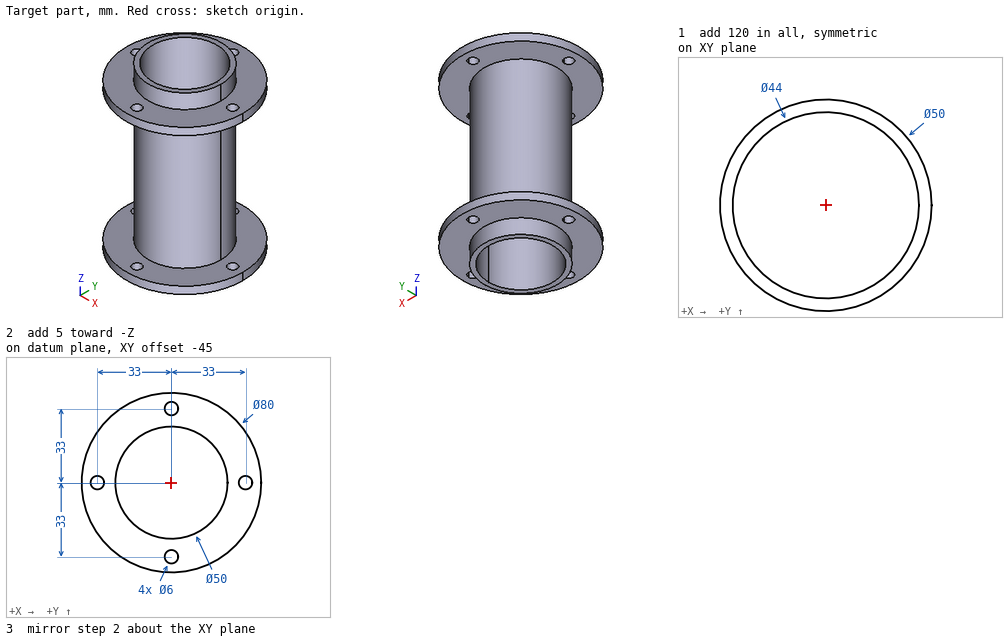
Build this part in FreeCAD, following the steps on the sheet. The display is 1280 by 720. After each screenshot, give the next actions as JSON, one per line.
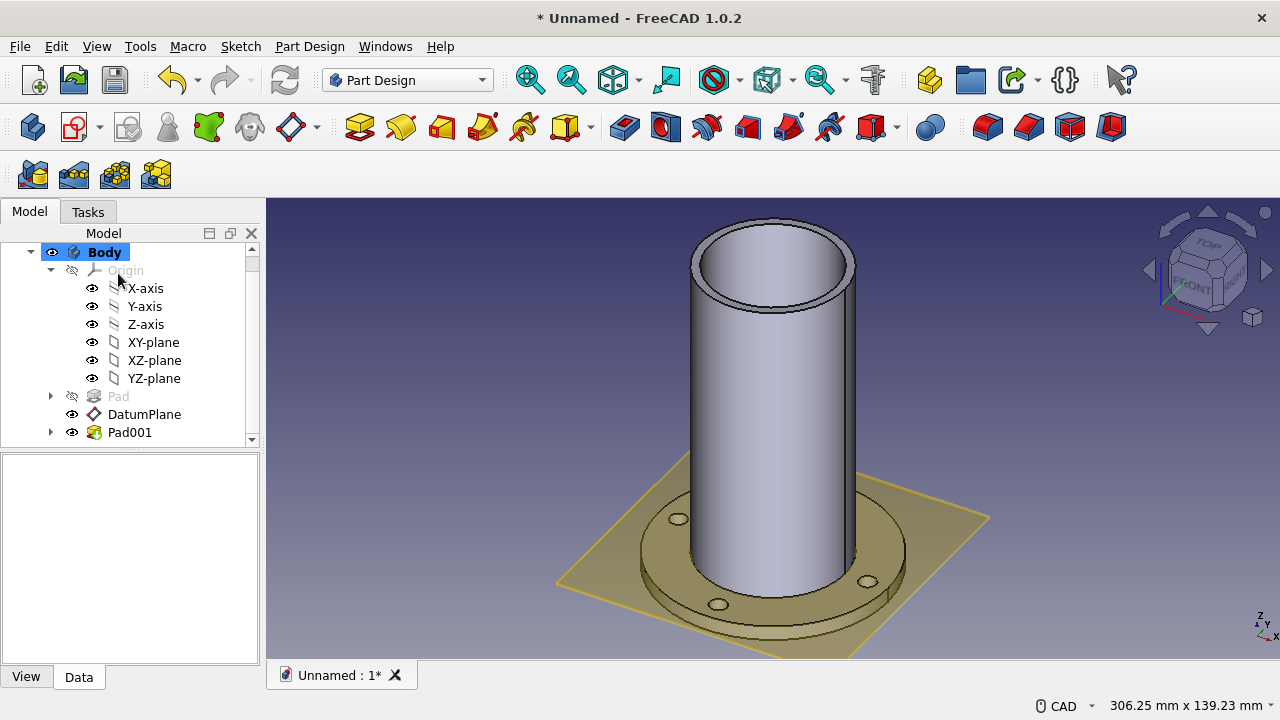
{"action": "left_click", "coordinate": [117, 414]}
{"action": "key", "text": "space"}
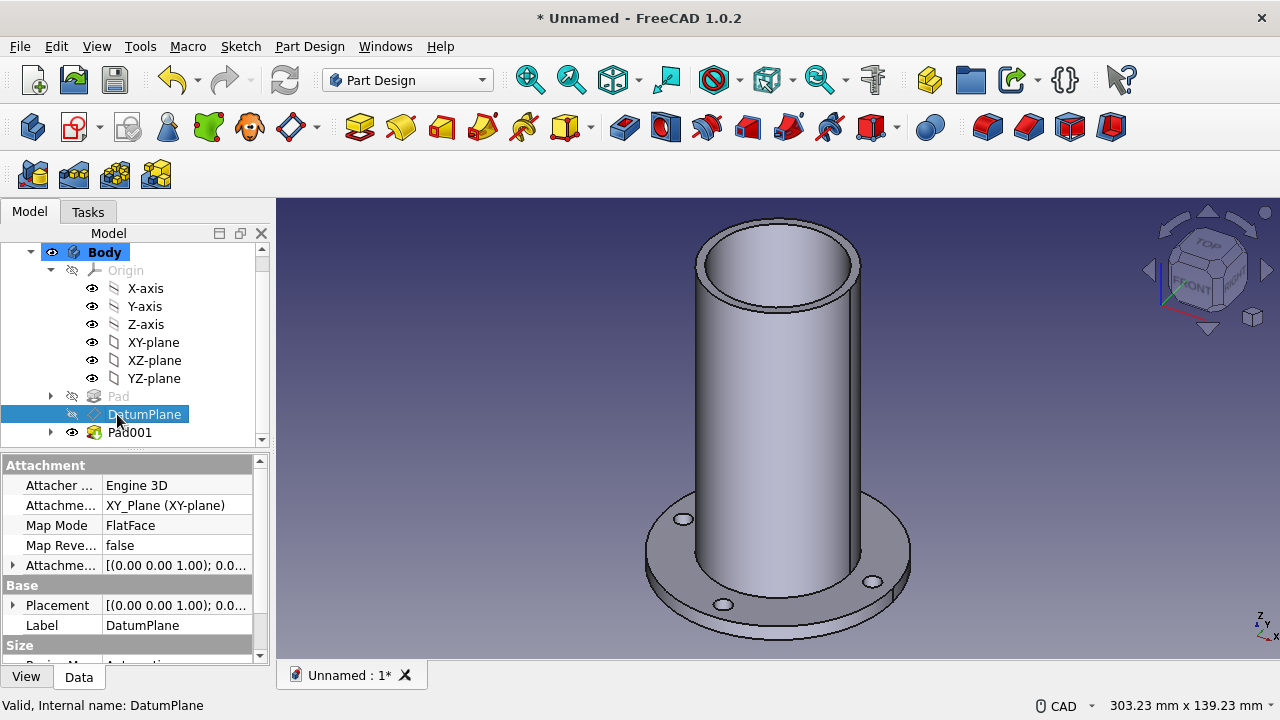
{"action": "left_click", "coordinate": [531, 80]}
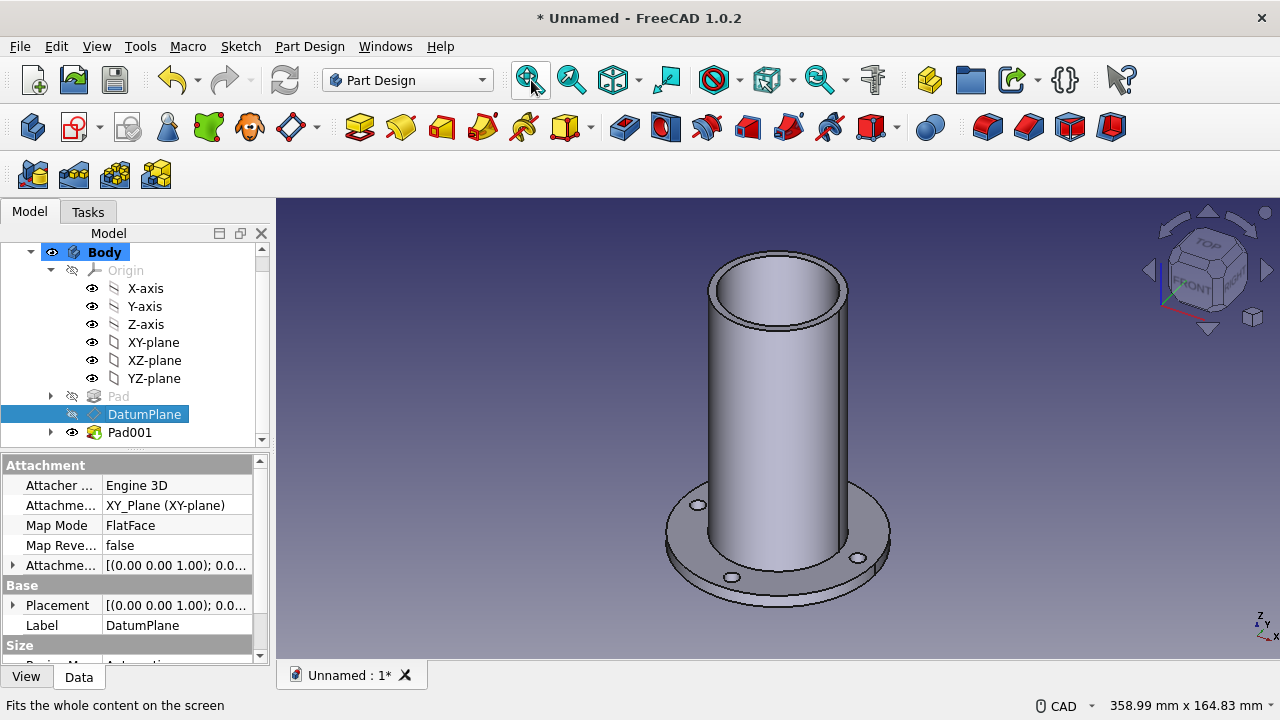
{"action": "left_click", "coordinate": [117, 432]}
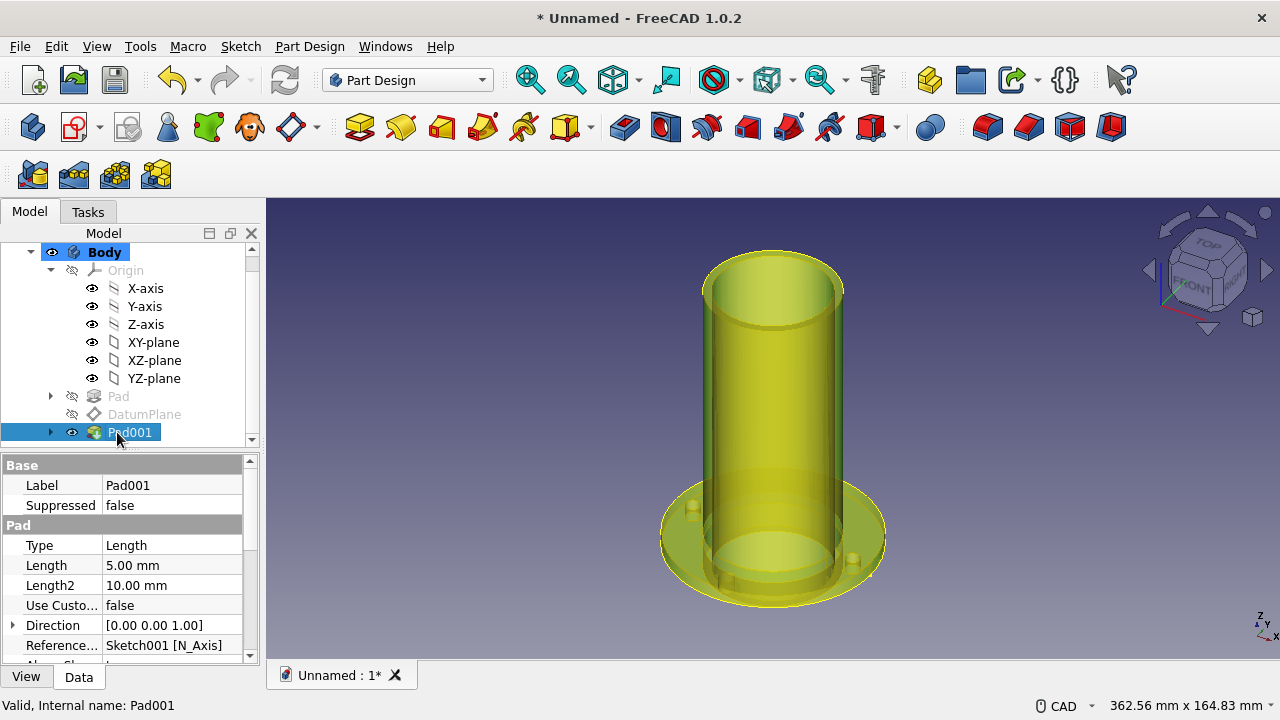
{"action": "left_click", "coordinate": [33, 174]}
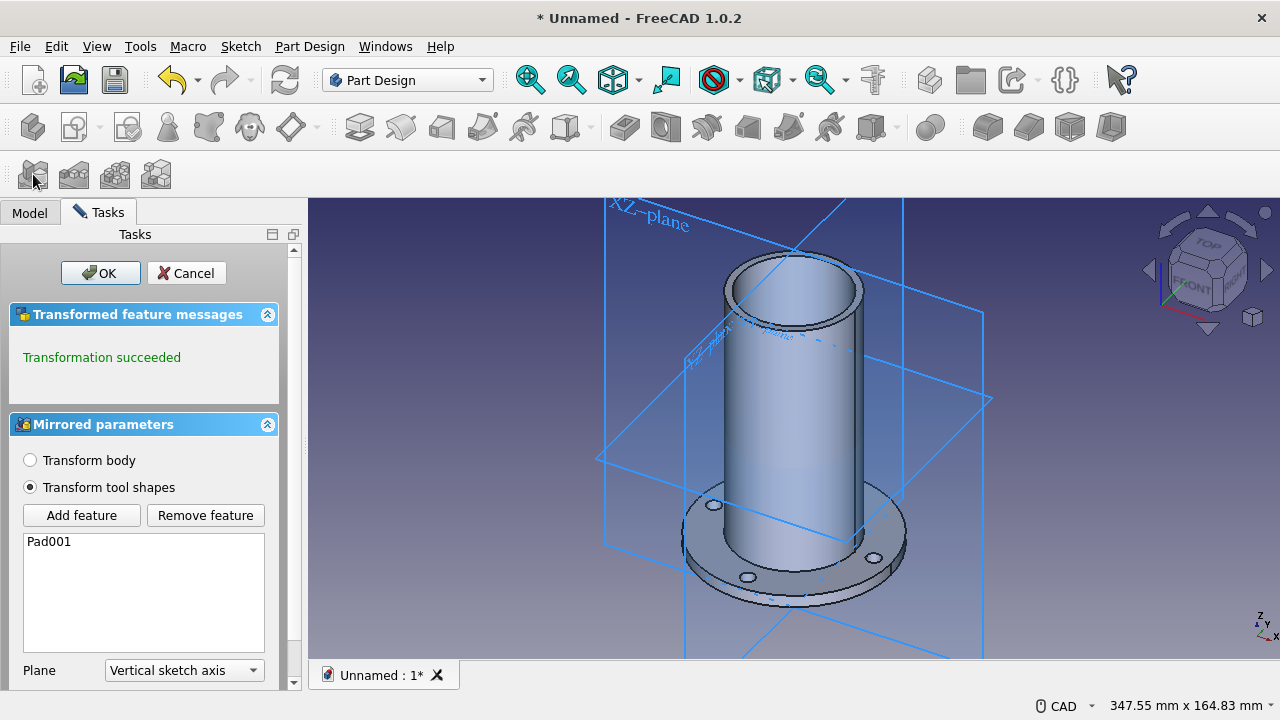
{"action": "left_click", "coordinate": [185, 670]}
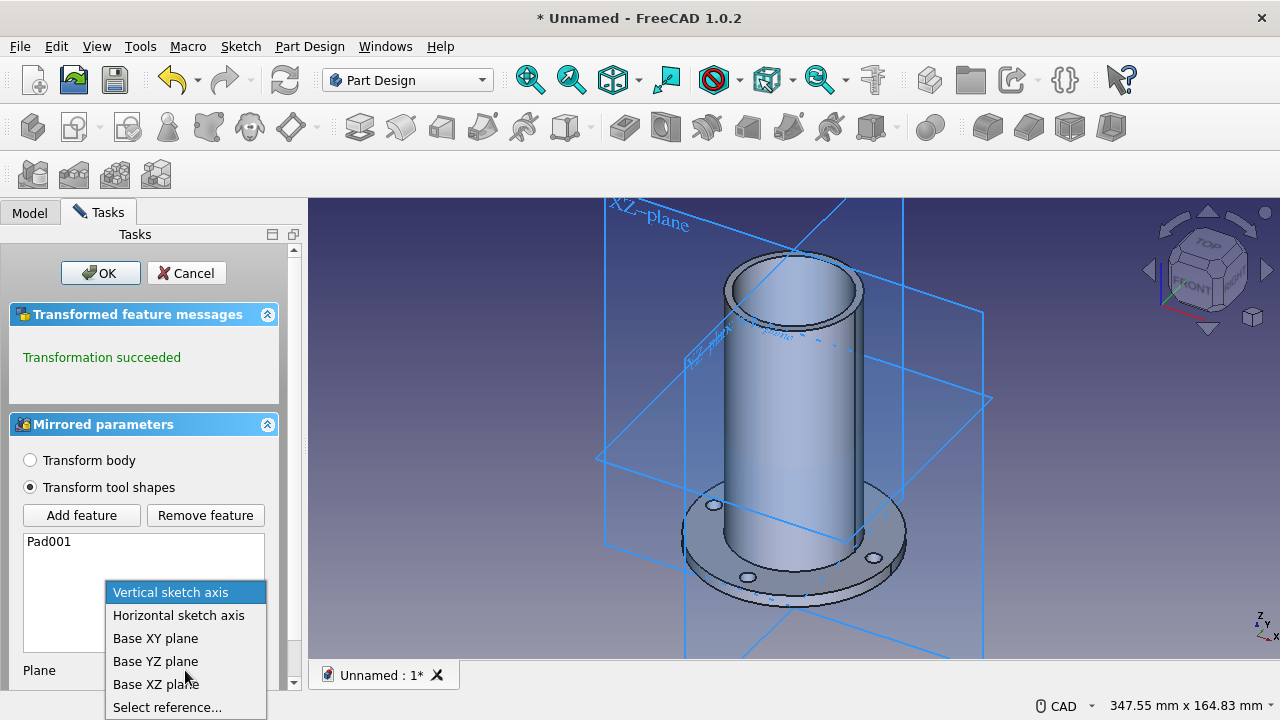
{"action": "left_click", "coordinate": [184, 638]}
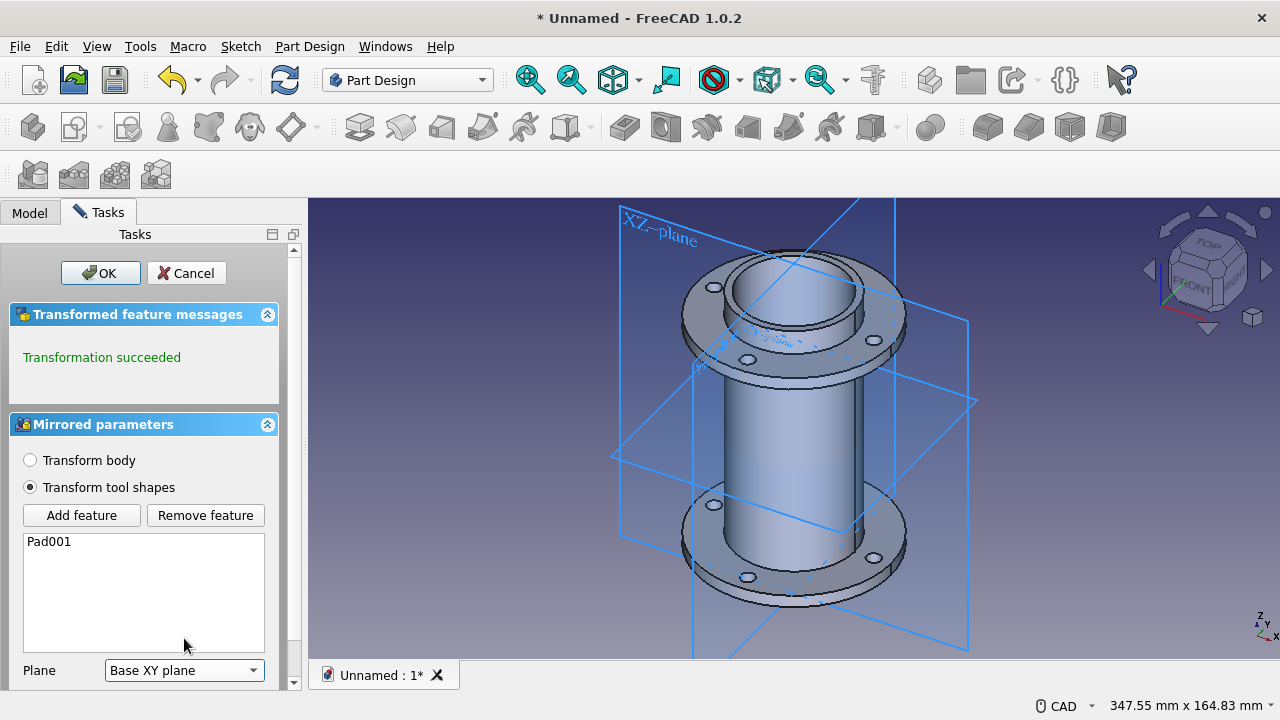
{"action": "left_click", "coordinate": [101, 273]}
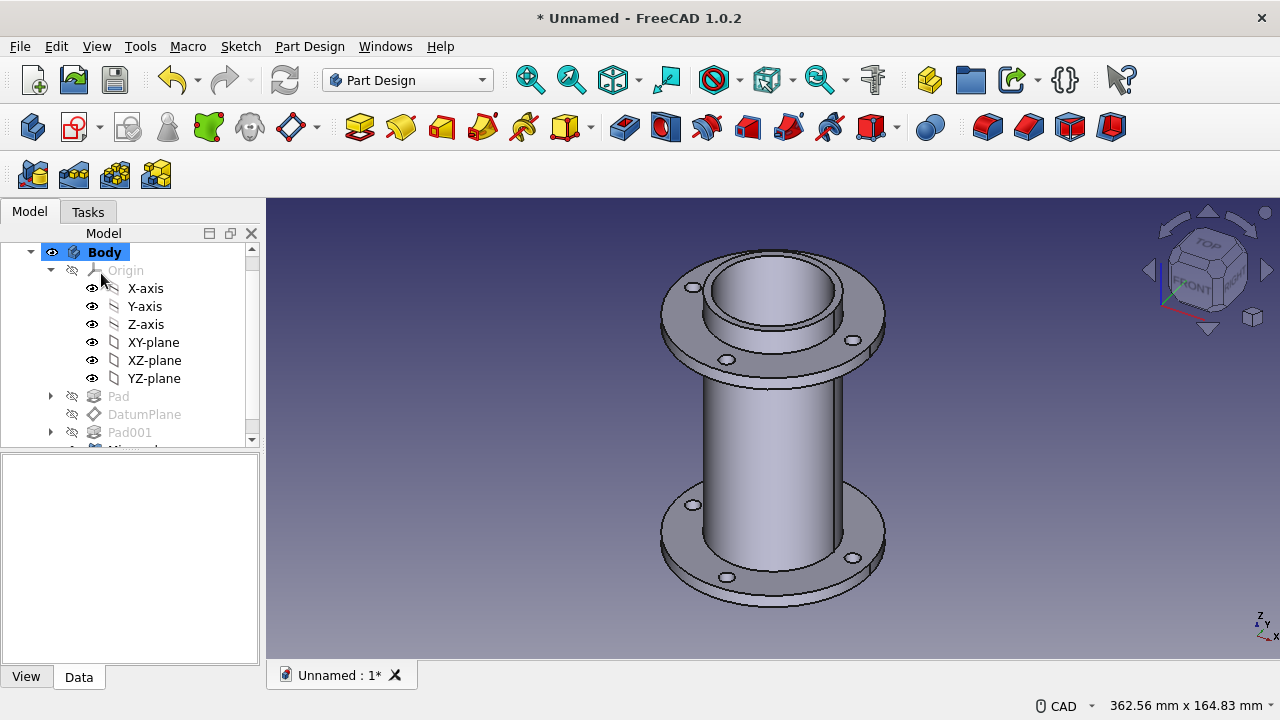
{"action": "key", "text": "0"}